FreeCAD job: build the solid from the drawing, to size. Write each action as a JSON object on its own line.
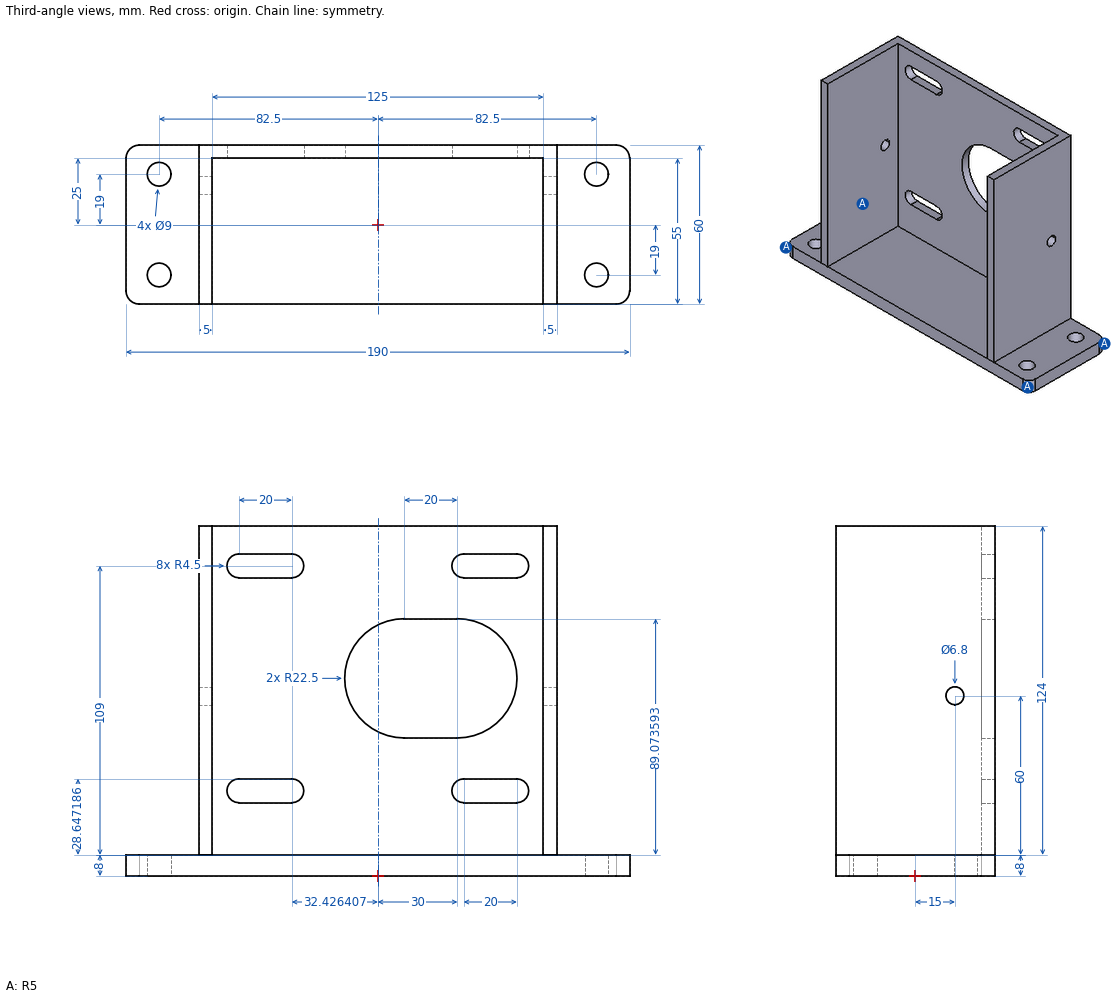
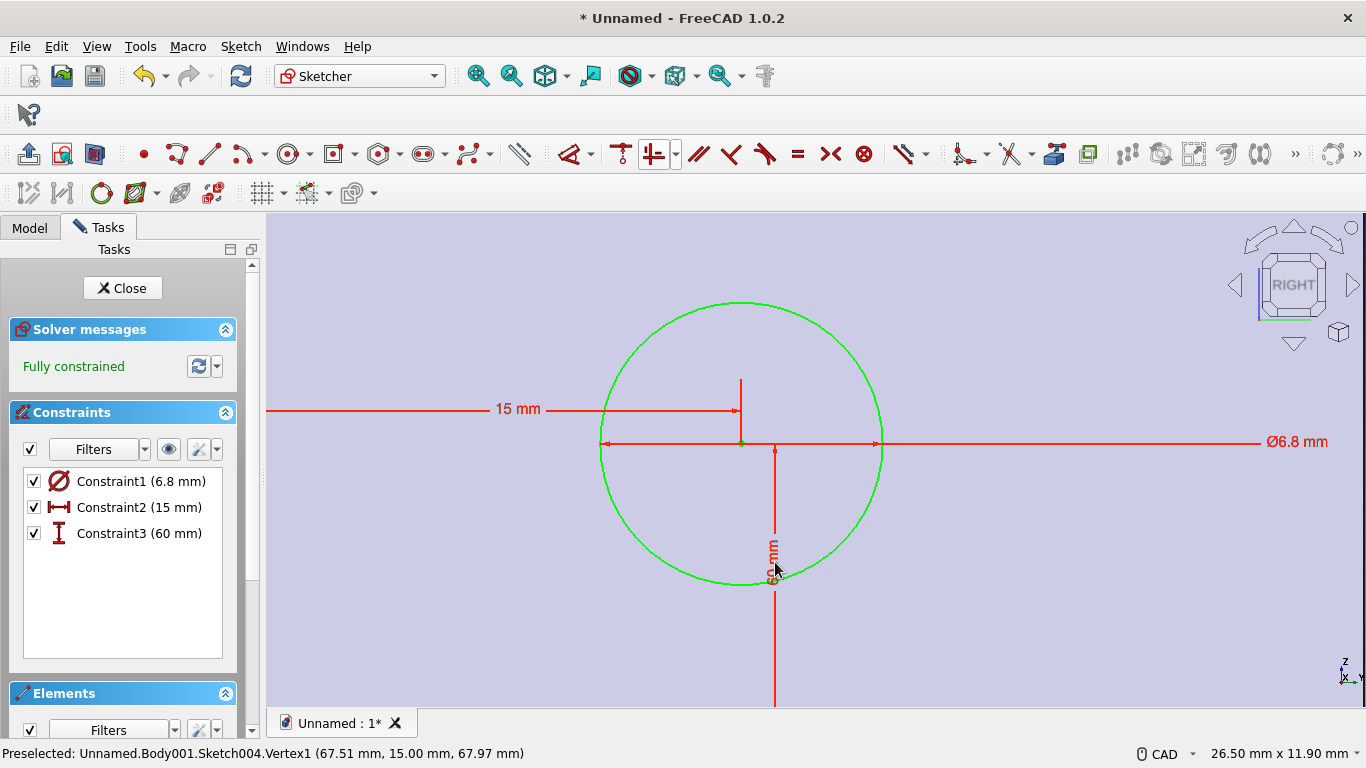
{"action": "left_click", "coordinate": [123, 288]}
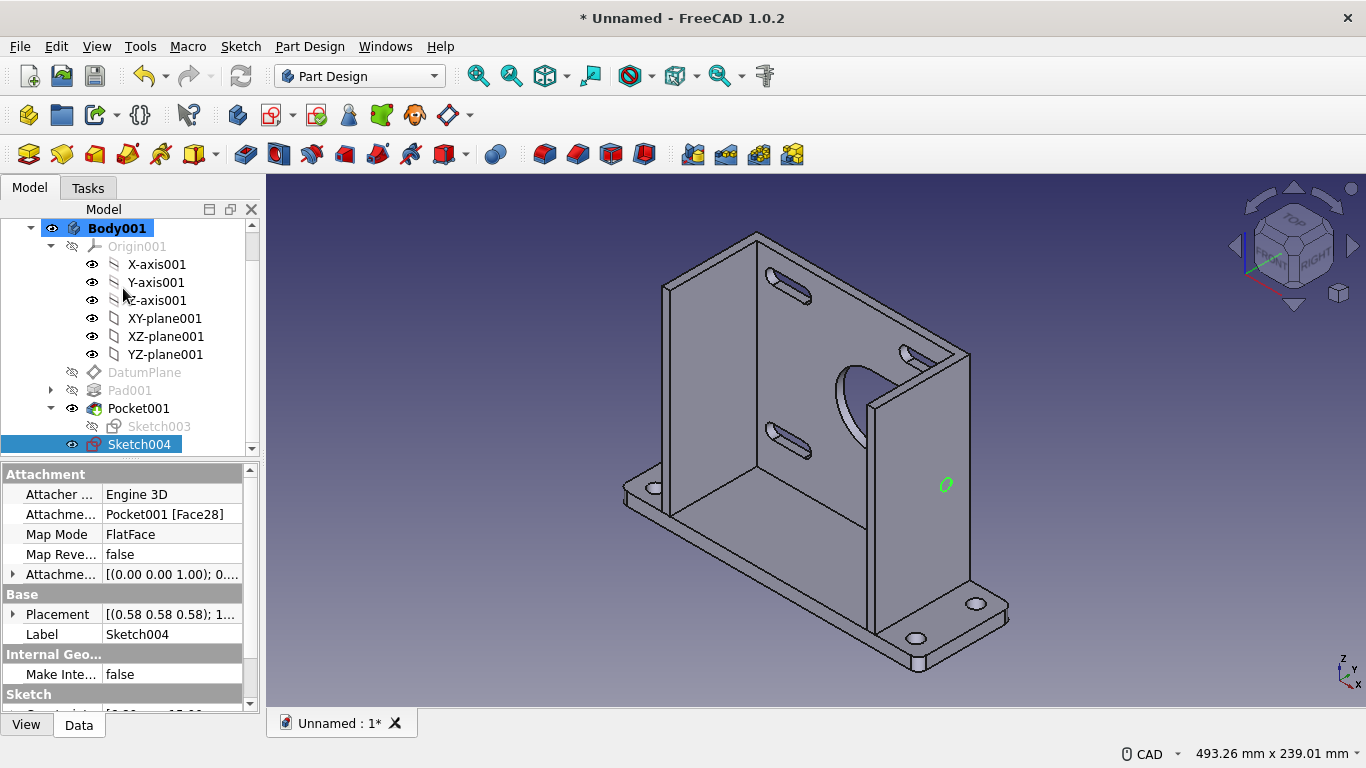
{"action": "left_click", "coordinate": [246, 154]}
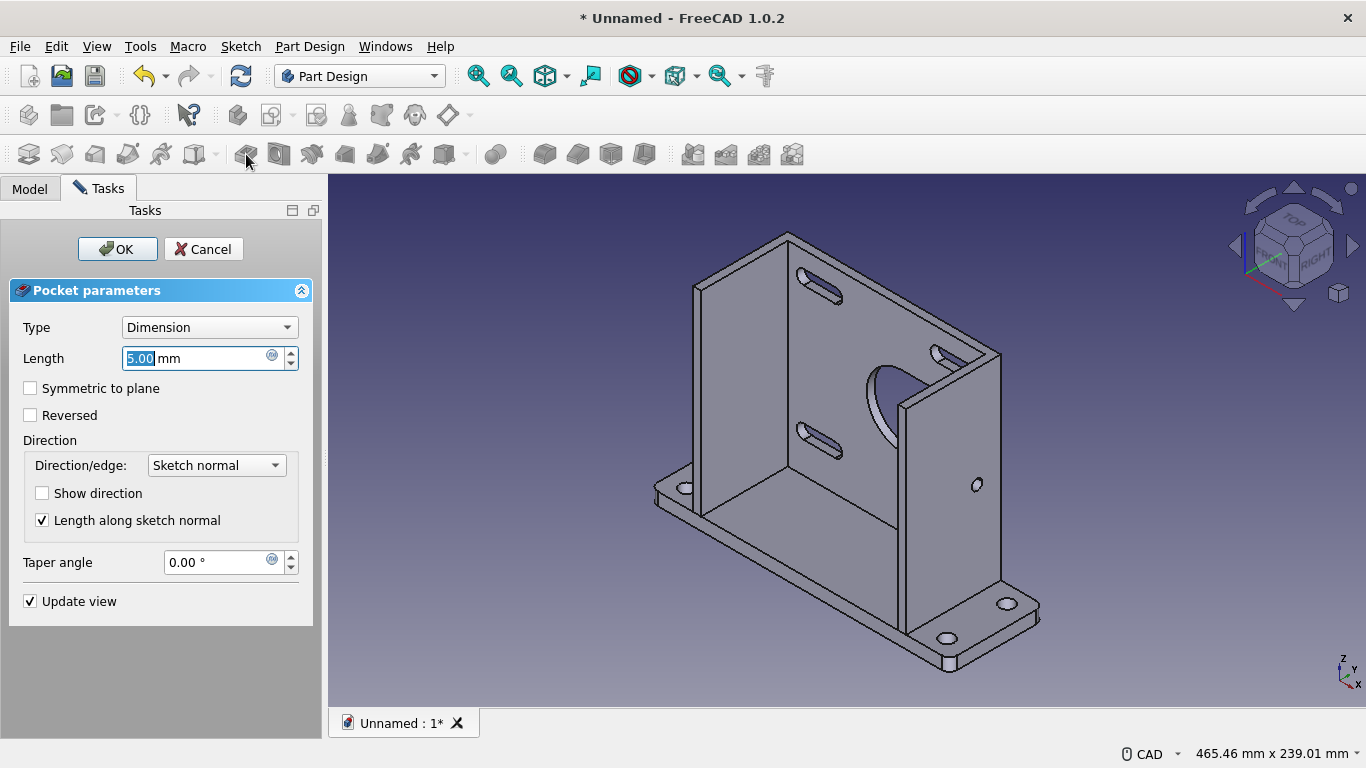
{"action": "left_click", "coordinate": [210, 328]}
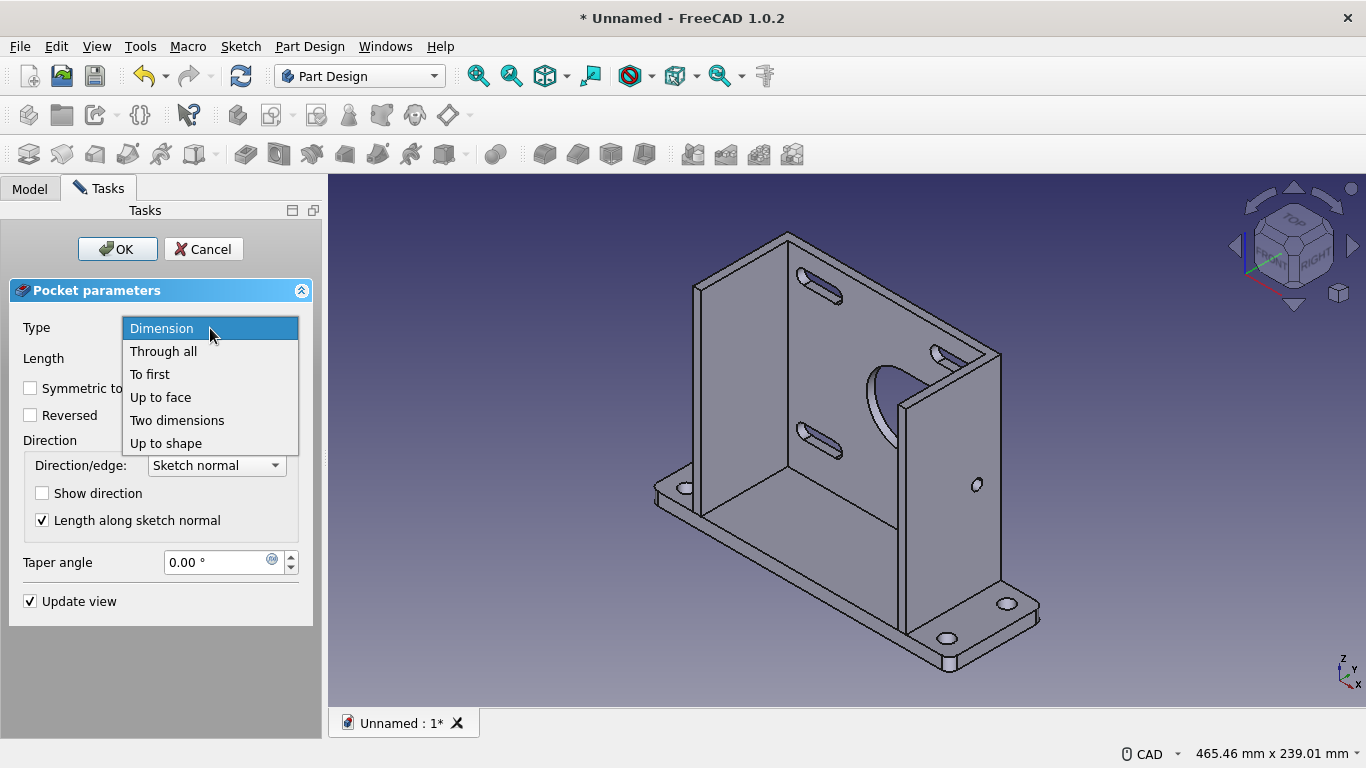
{"action": "left_click", "coordinate": [208, 352]}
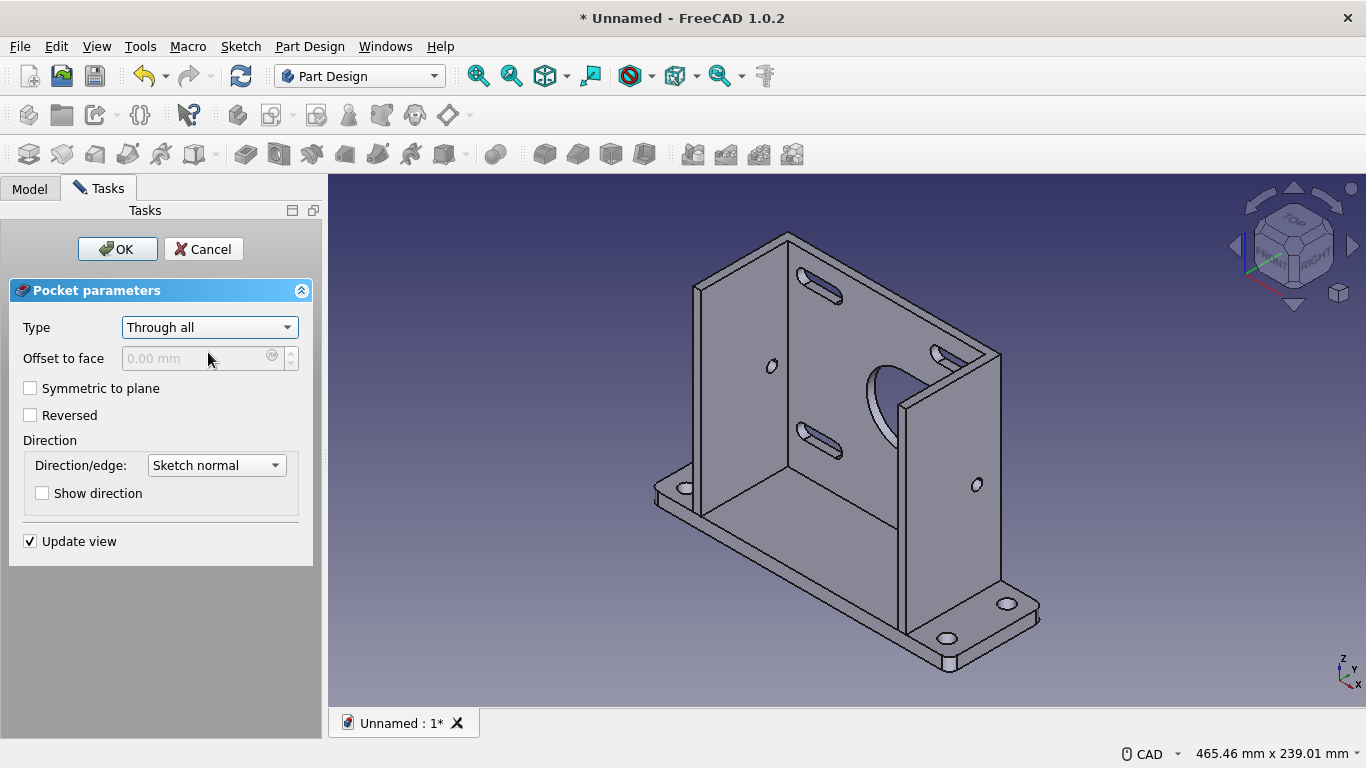
{"action": "left_click", "coordinate": [118, 249]}